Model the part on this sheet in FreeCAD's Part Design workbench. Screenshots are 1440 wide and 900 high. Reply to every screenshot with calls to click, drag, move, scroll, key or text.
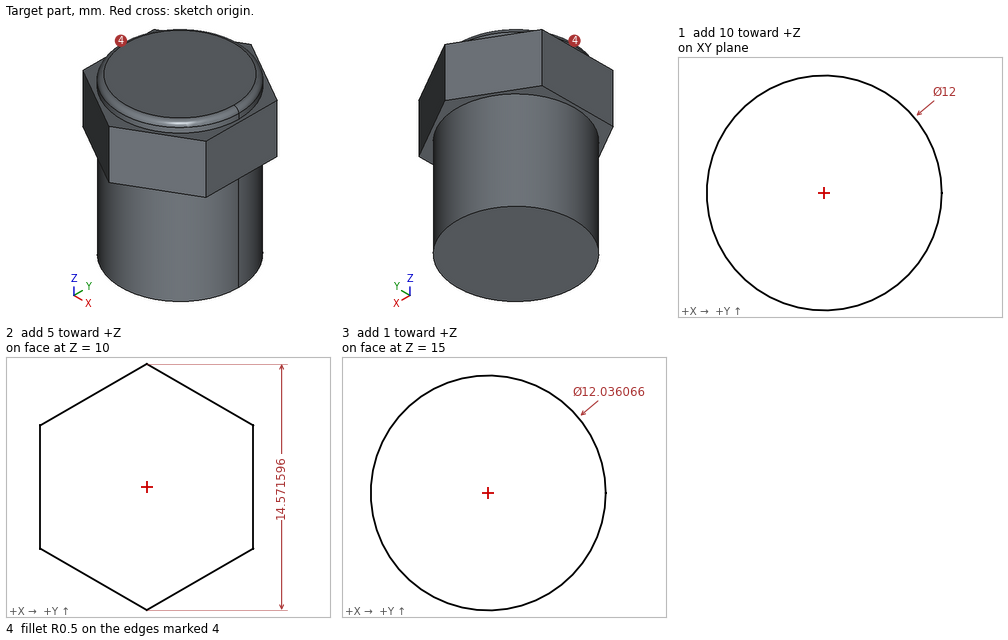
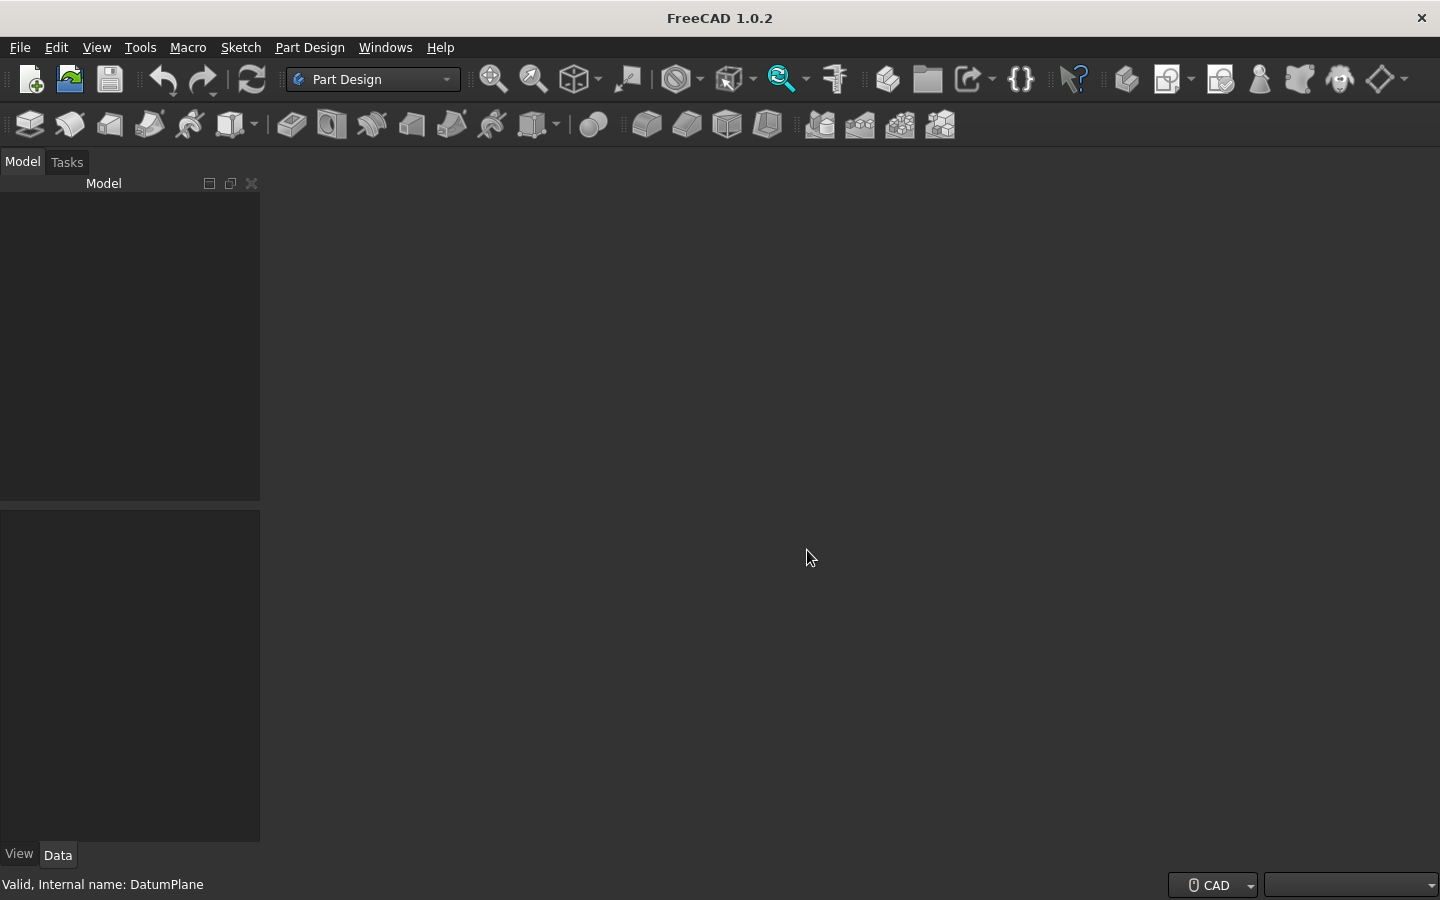
click(30, 80)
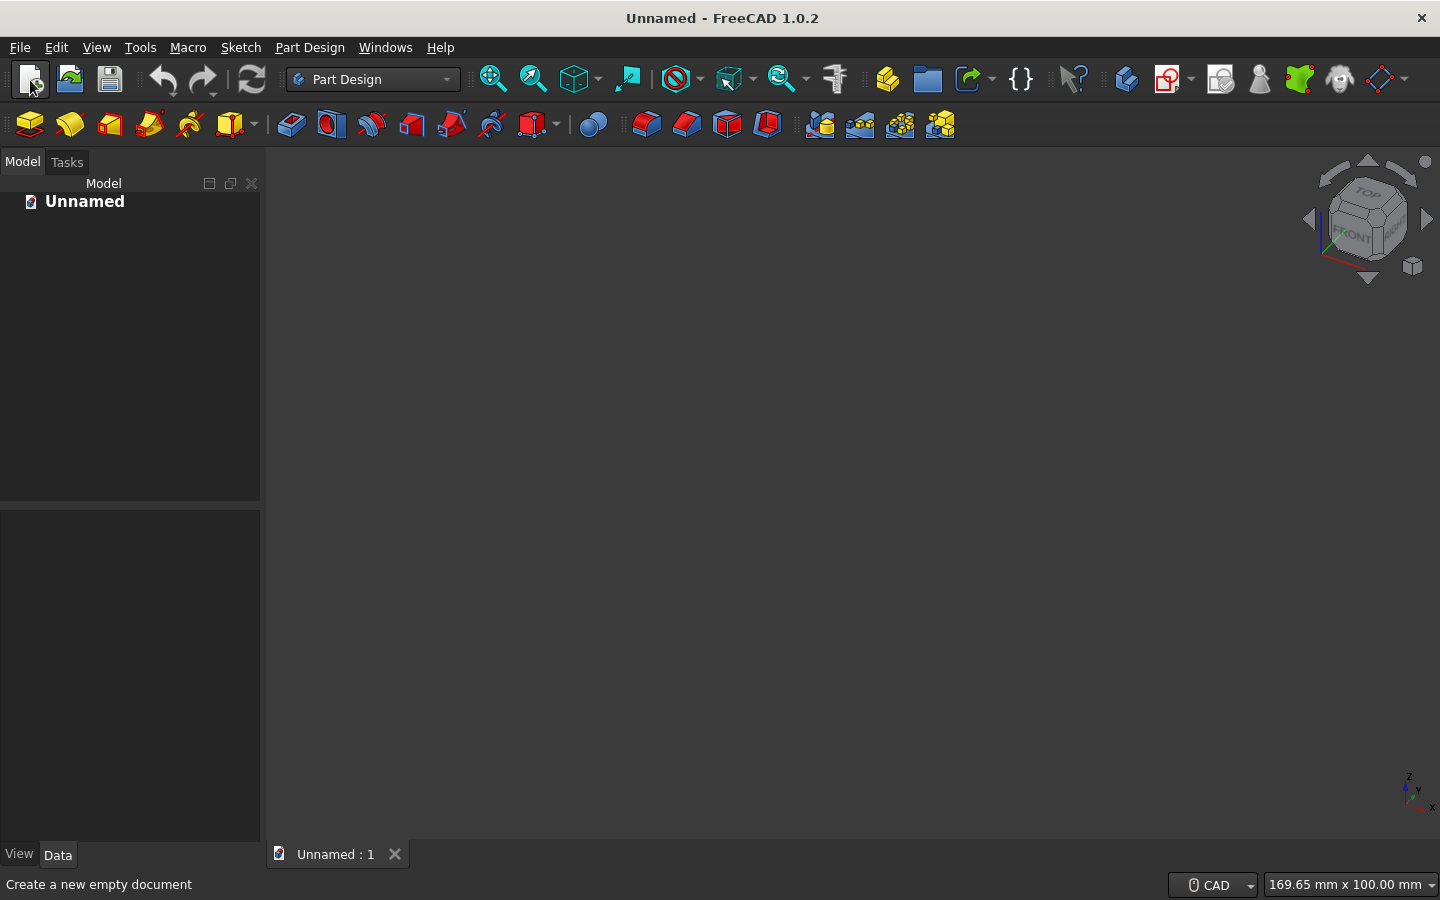
click(1168, 80)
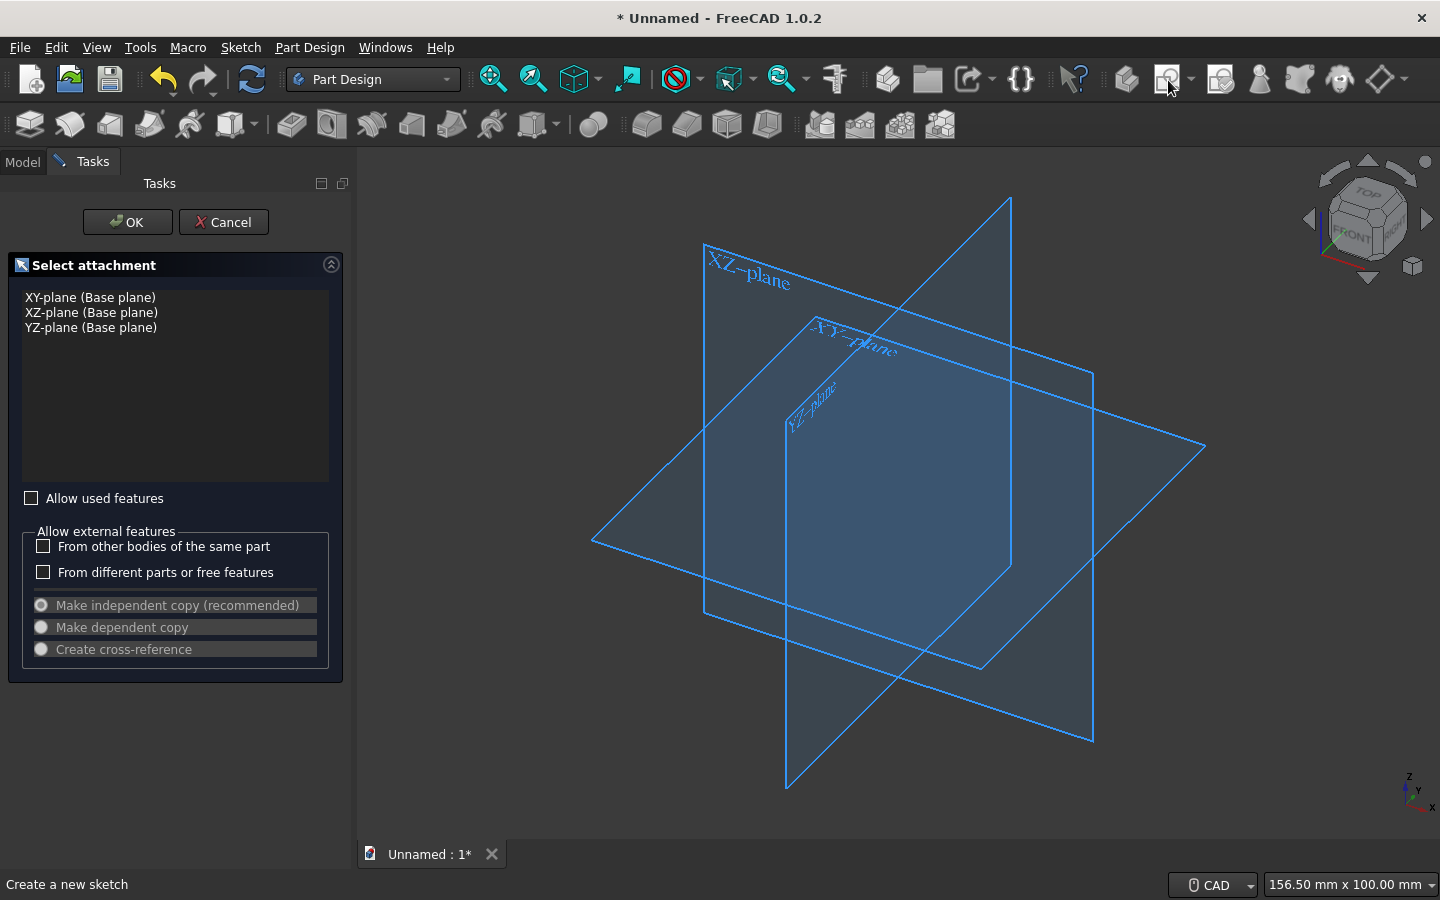
click(82, 298)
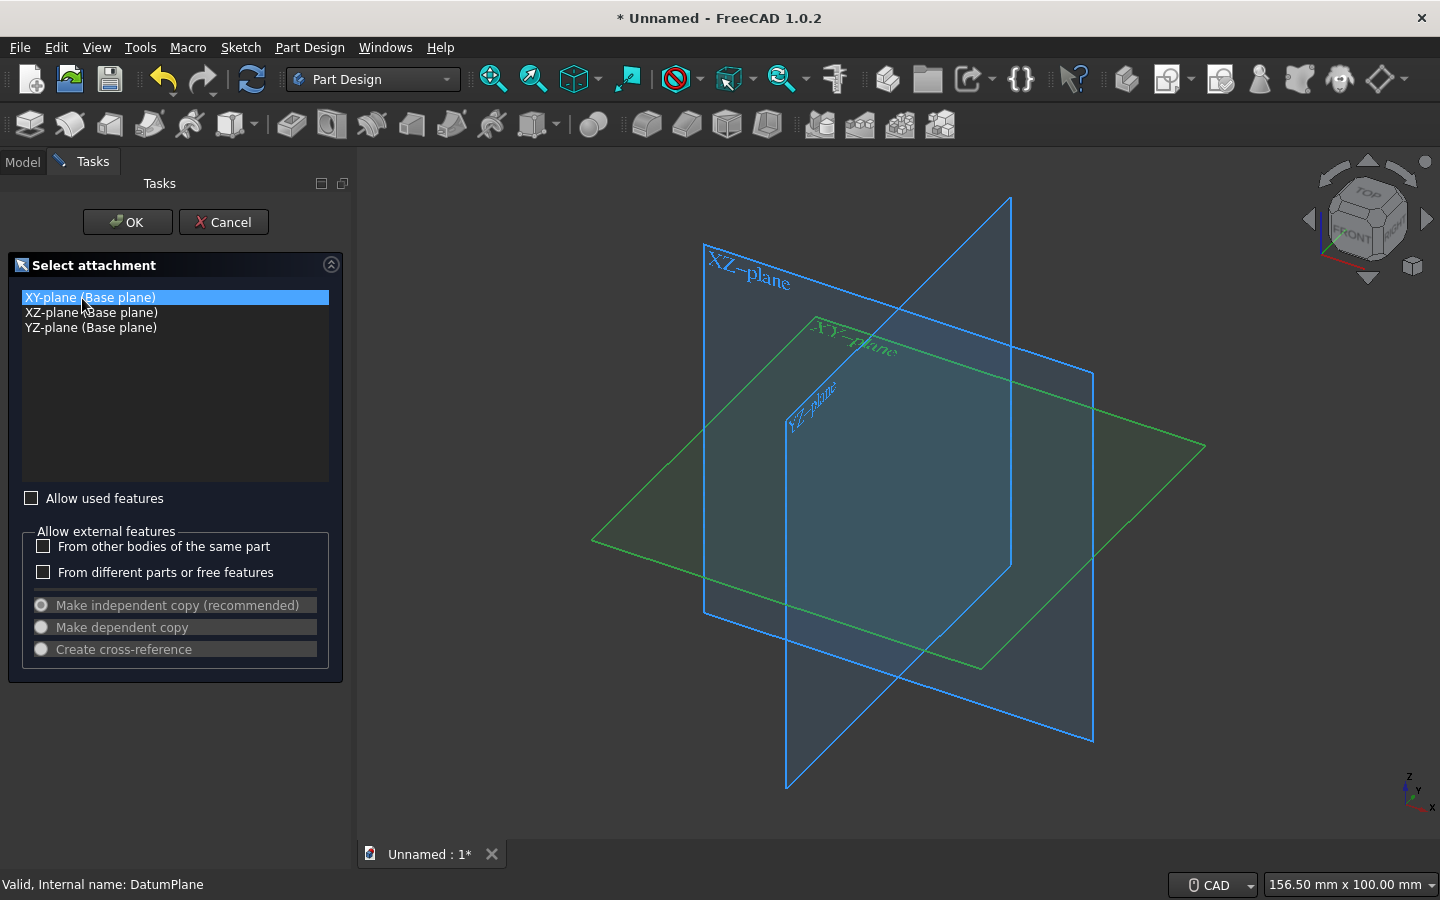
click(128, 222)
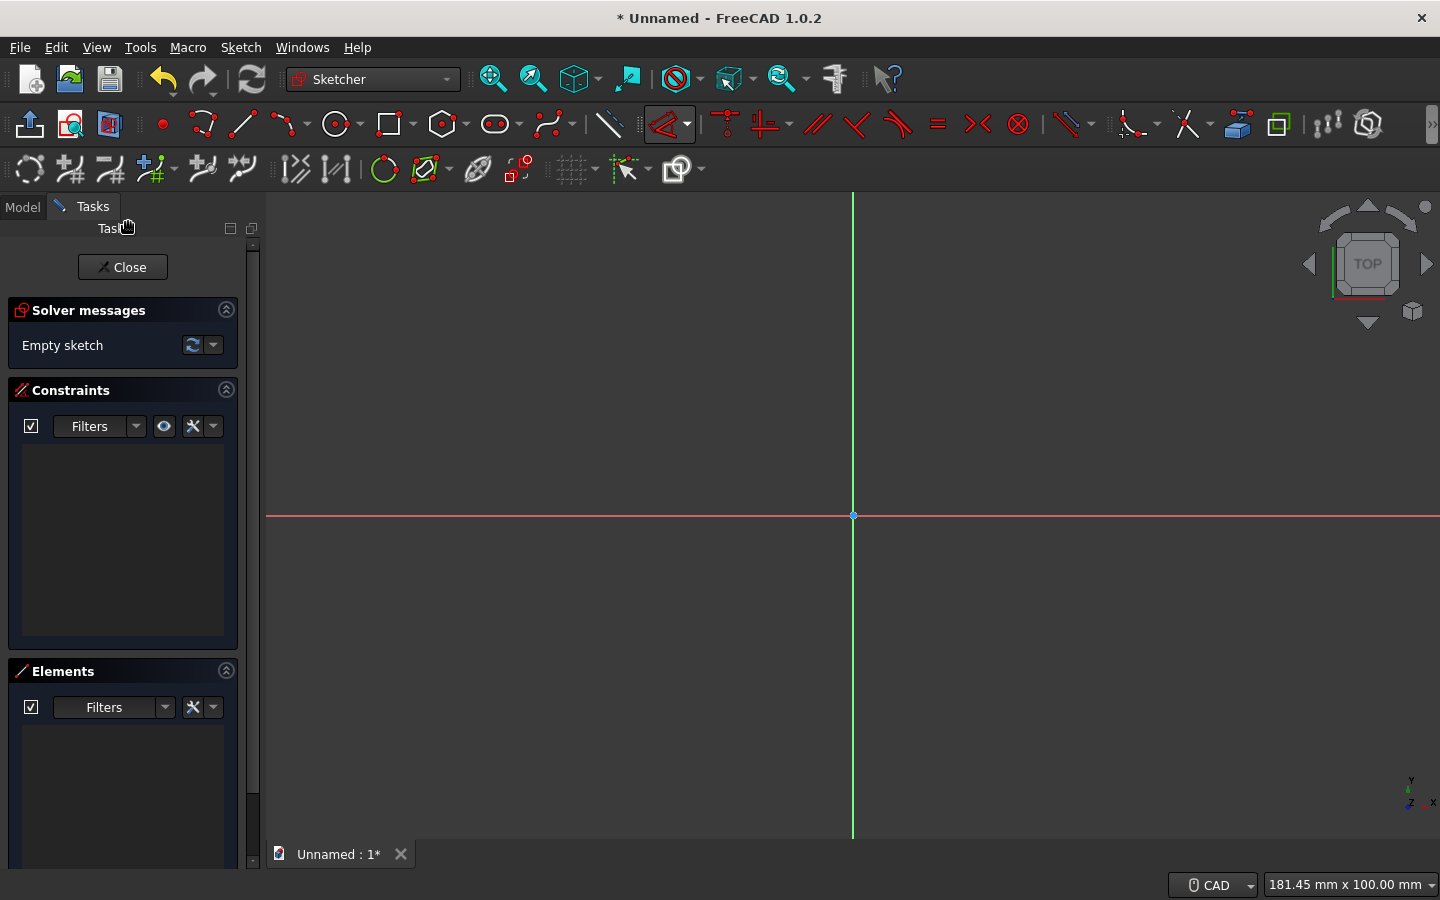
scroll(870, 516, up, 8)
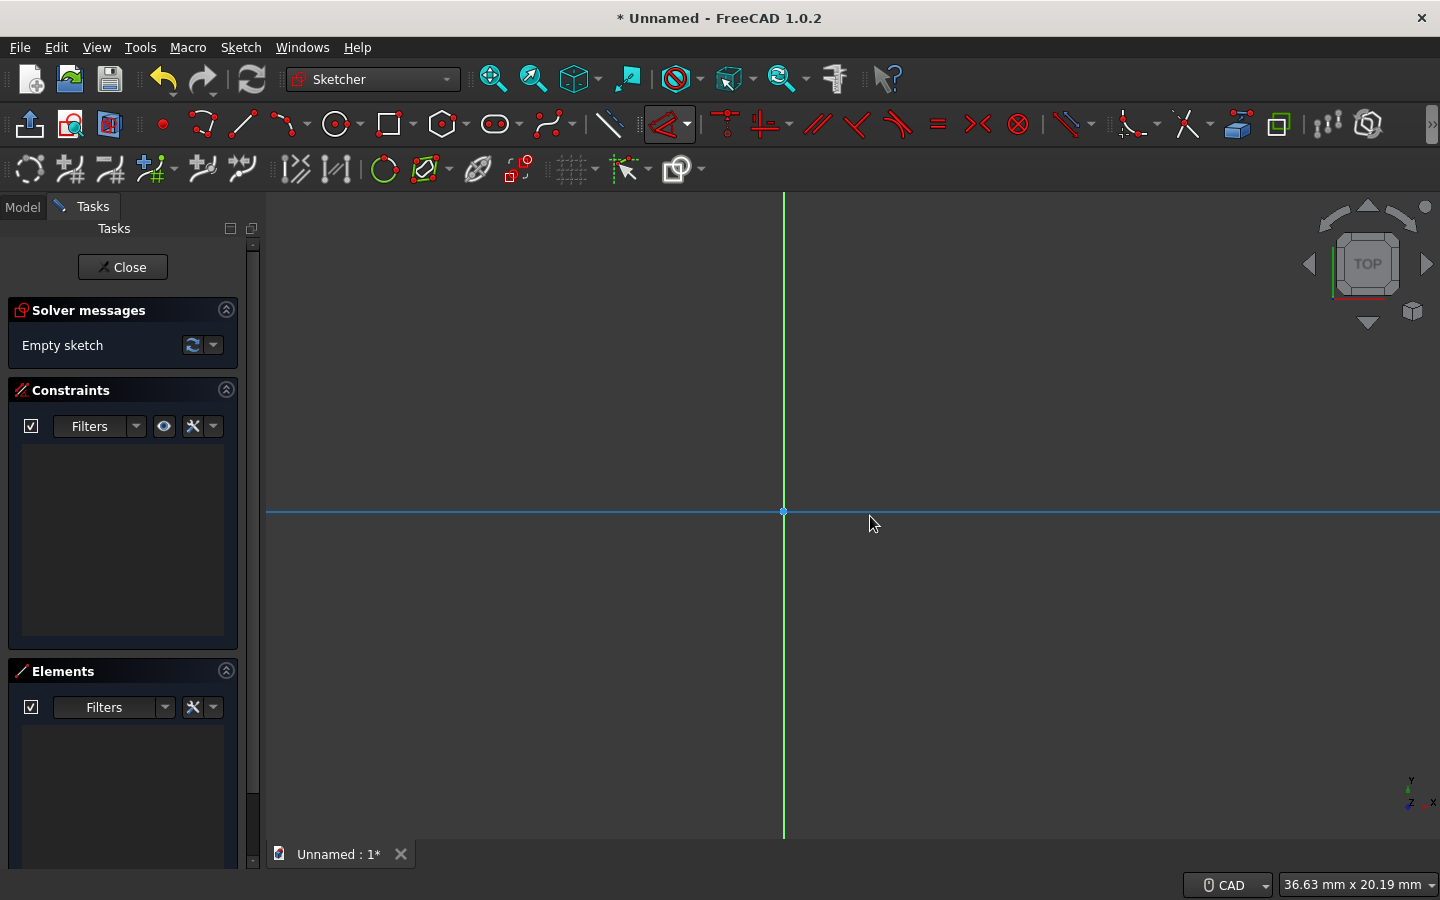
click(336, 124)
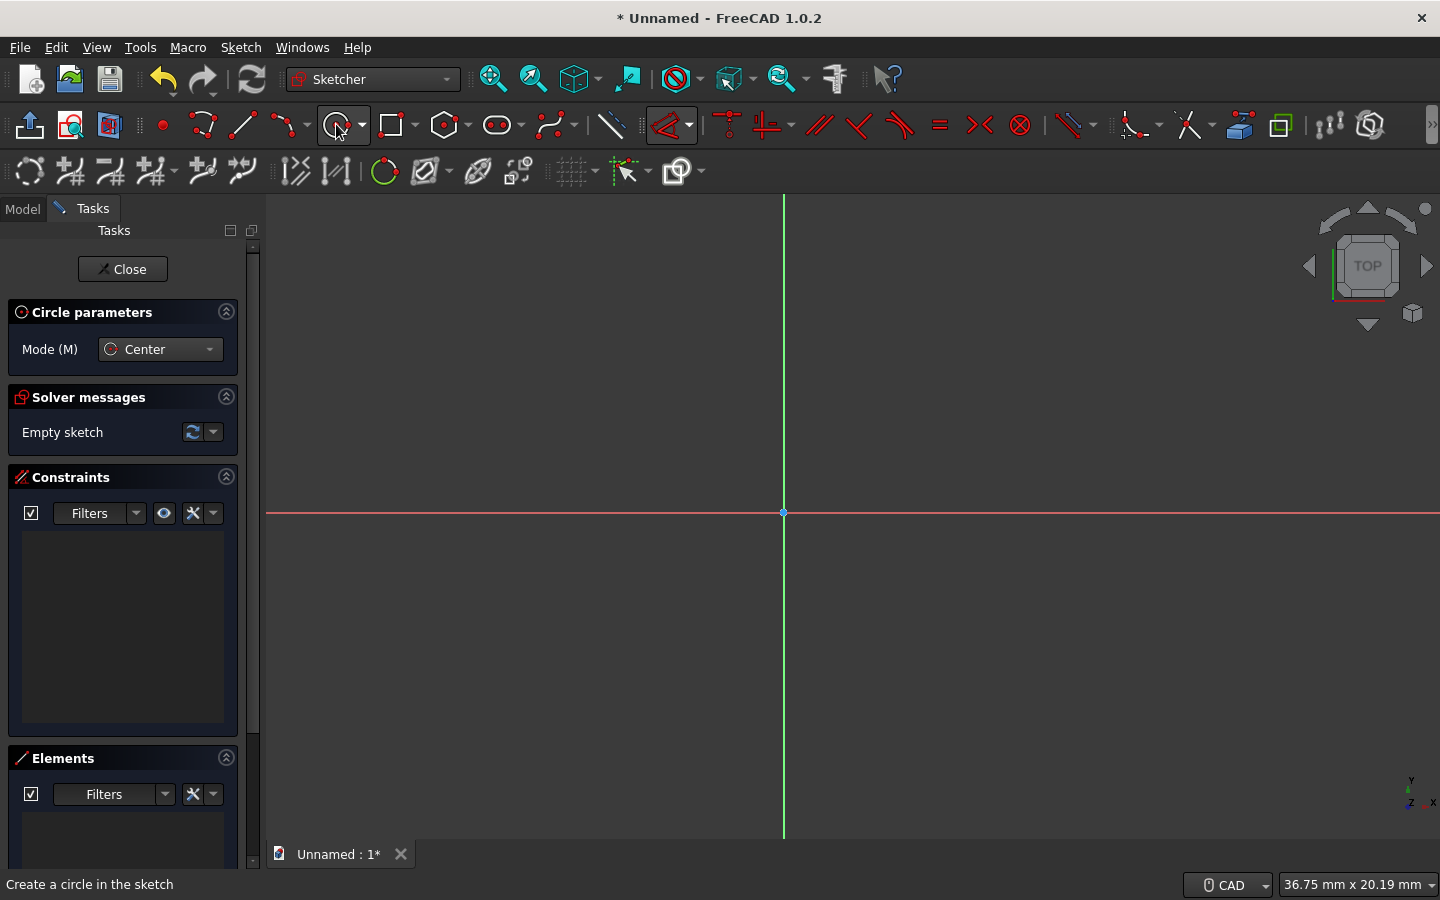
click(784, 513)
click(920, 377)
key(Escape)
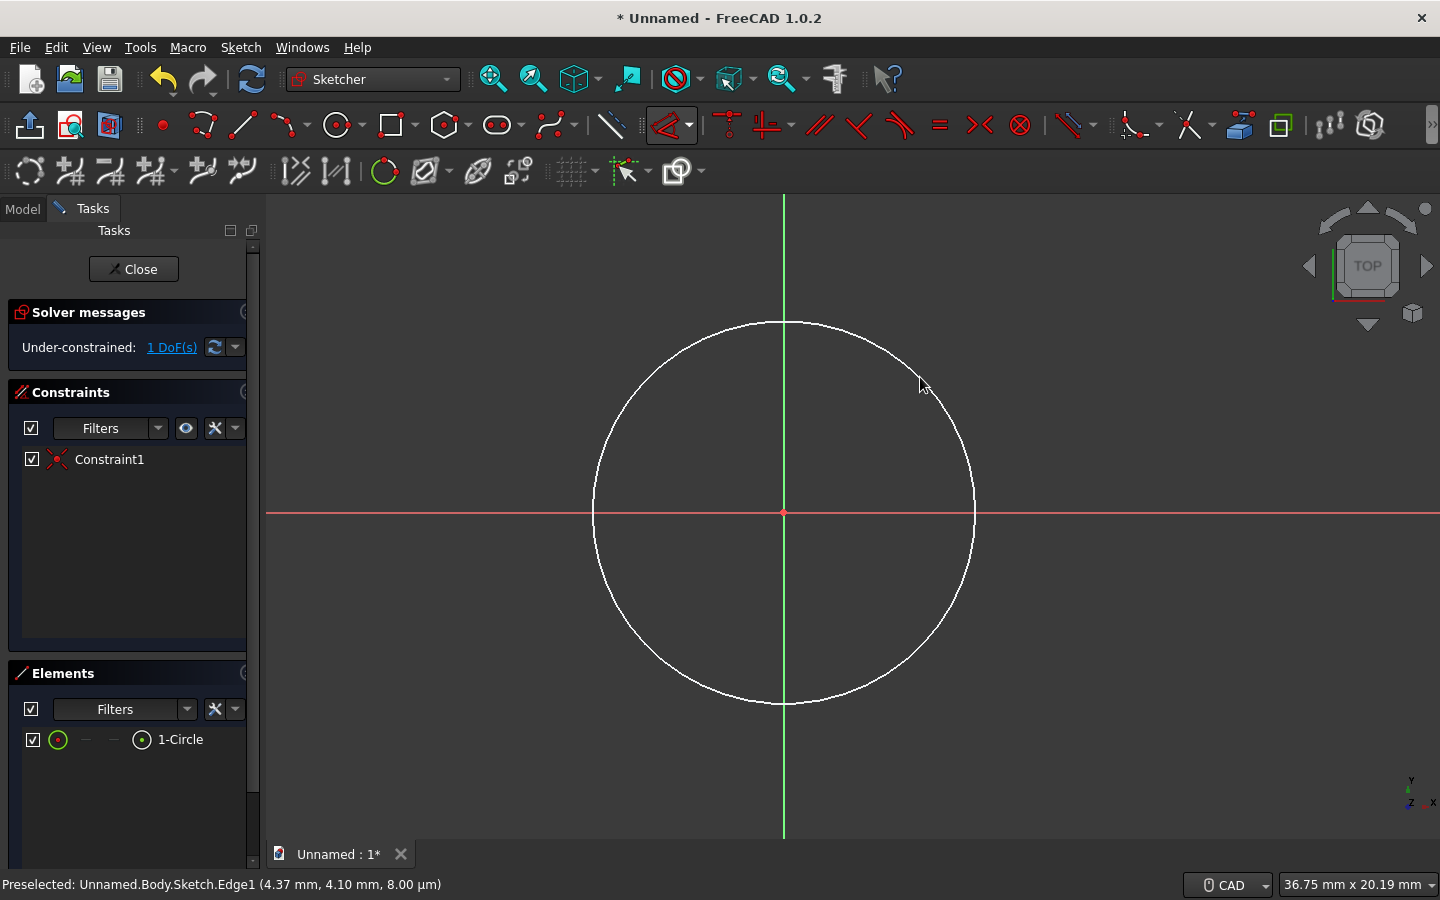
click(919, 377)